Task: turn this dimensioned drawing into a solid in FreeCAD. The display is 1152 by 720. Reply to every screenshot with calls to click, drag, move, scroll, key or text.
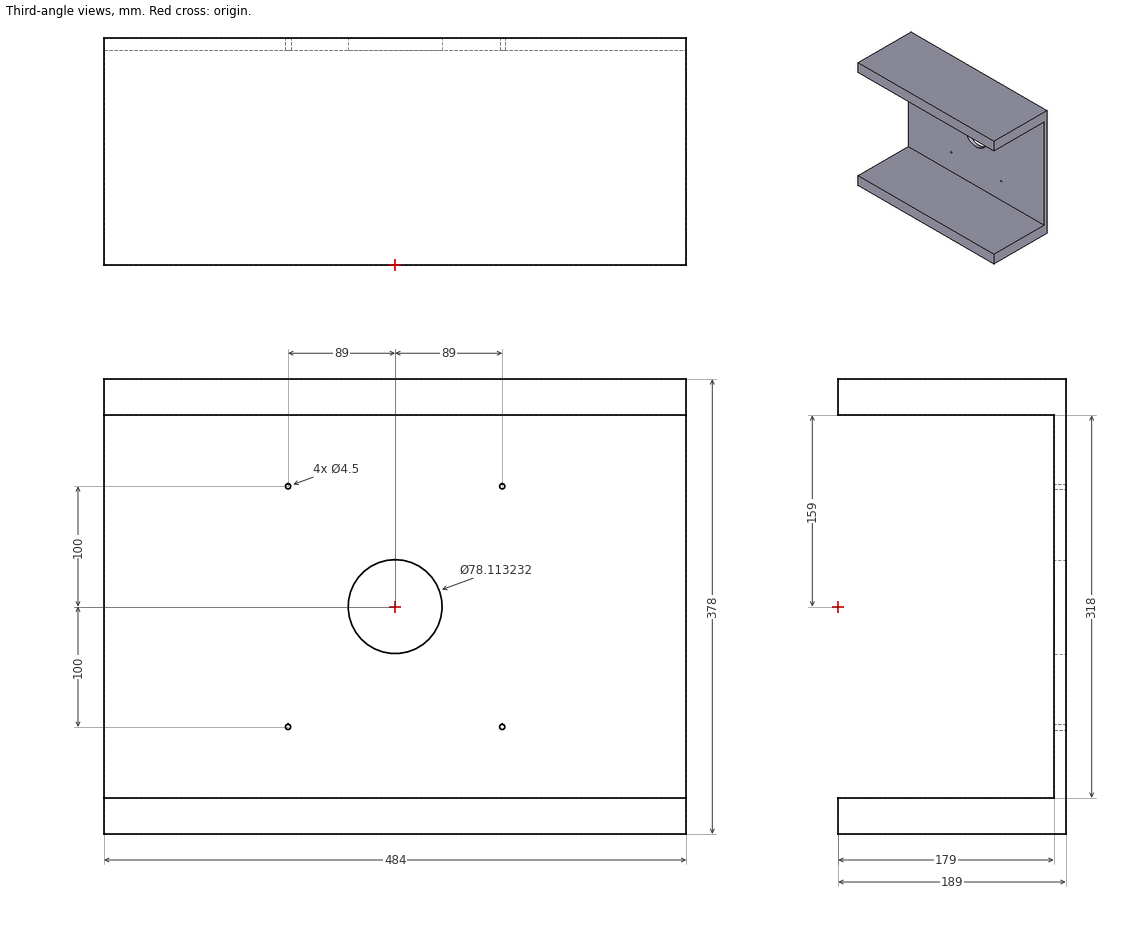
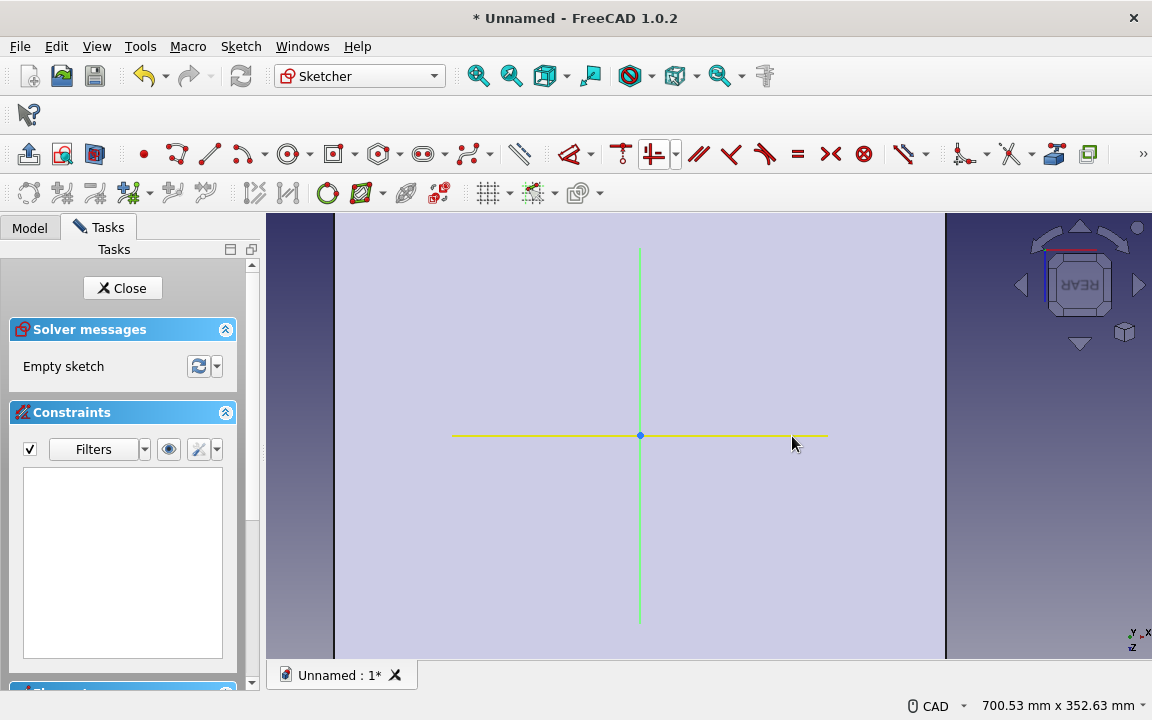
click(288, 154)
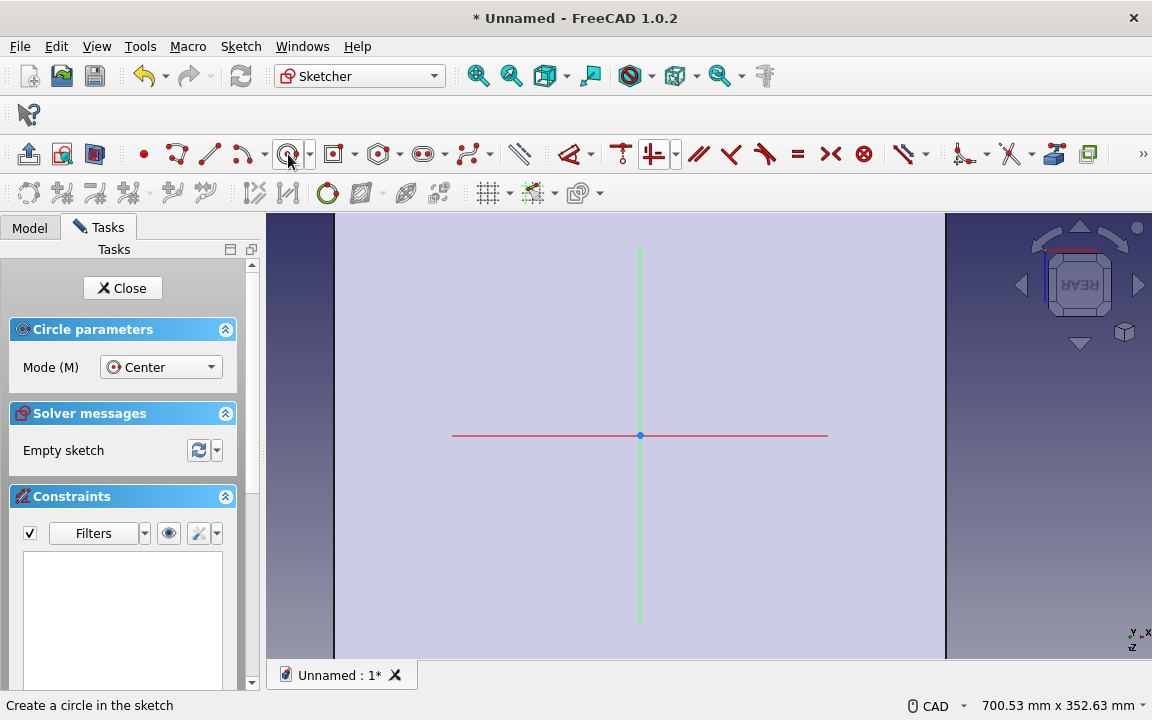
scroll(528, 562, up, 11)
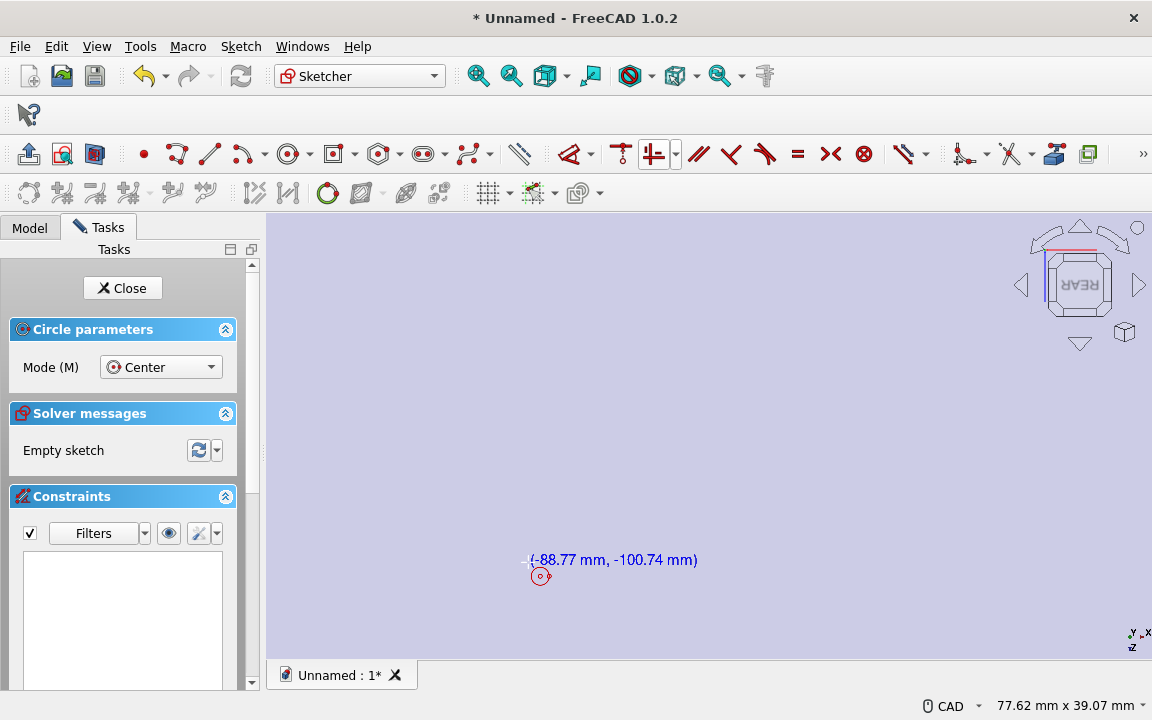
scroll(529, 563, down, 11)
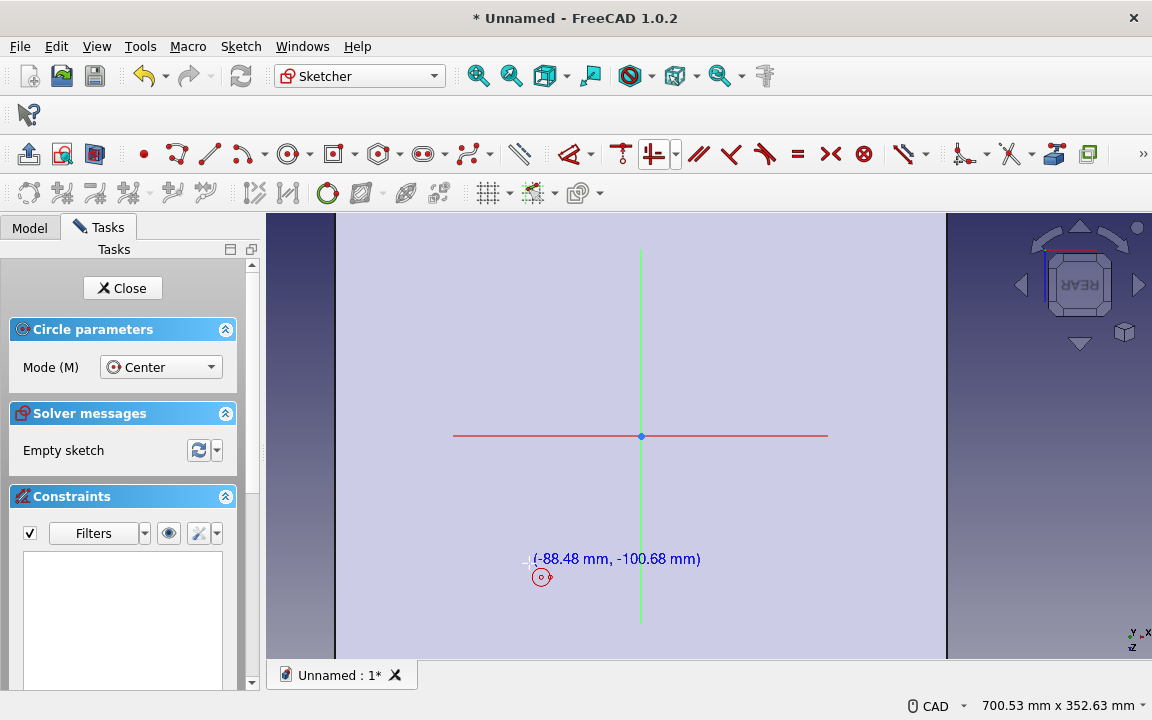
click(529, 563)
move(531, 561)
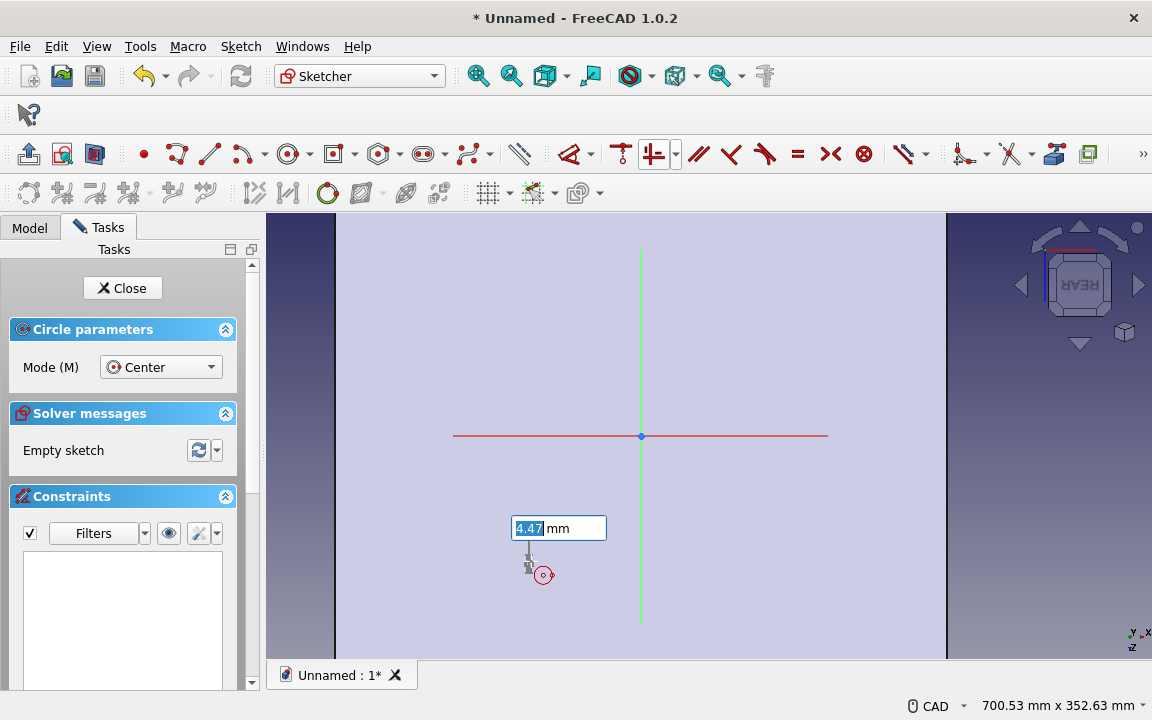
text(4.5)
key(Return)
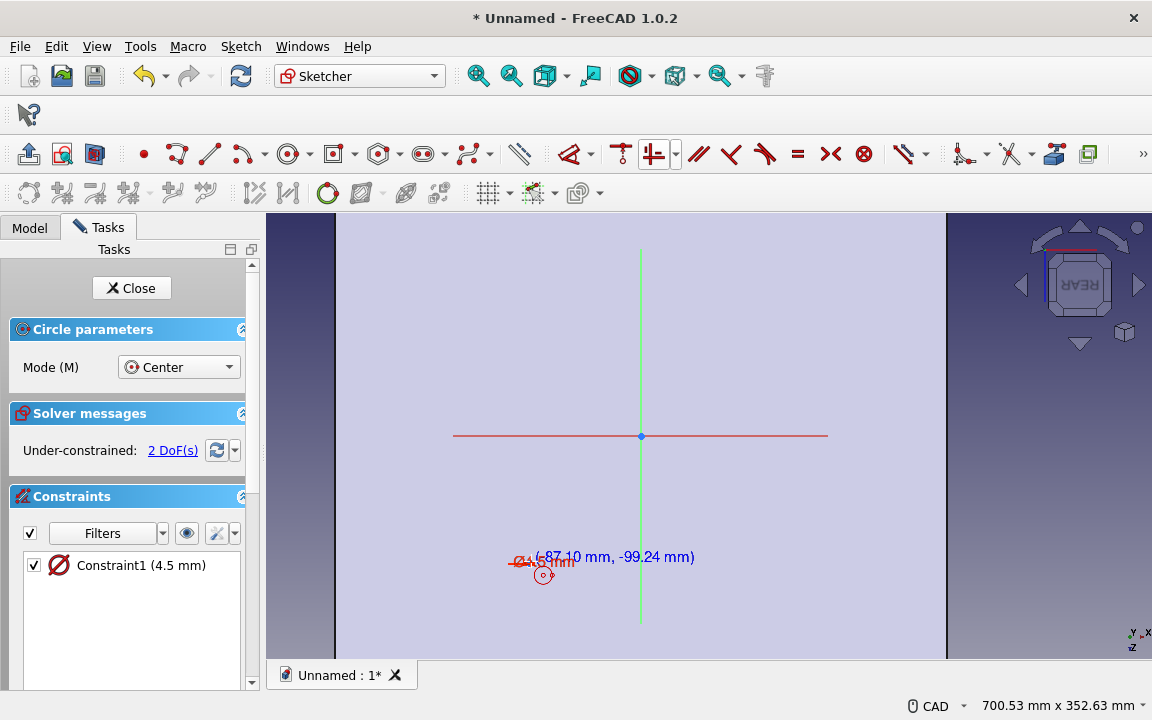
scroll(754, 563, up, 11)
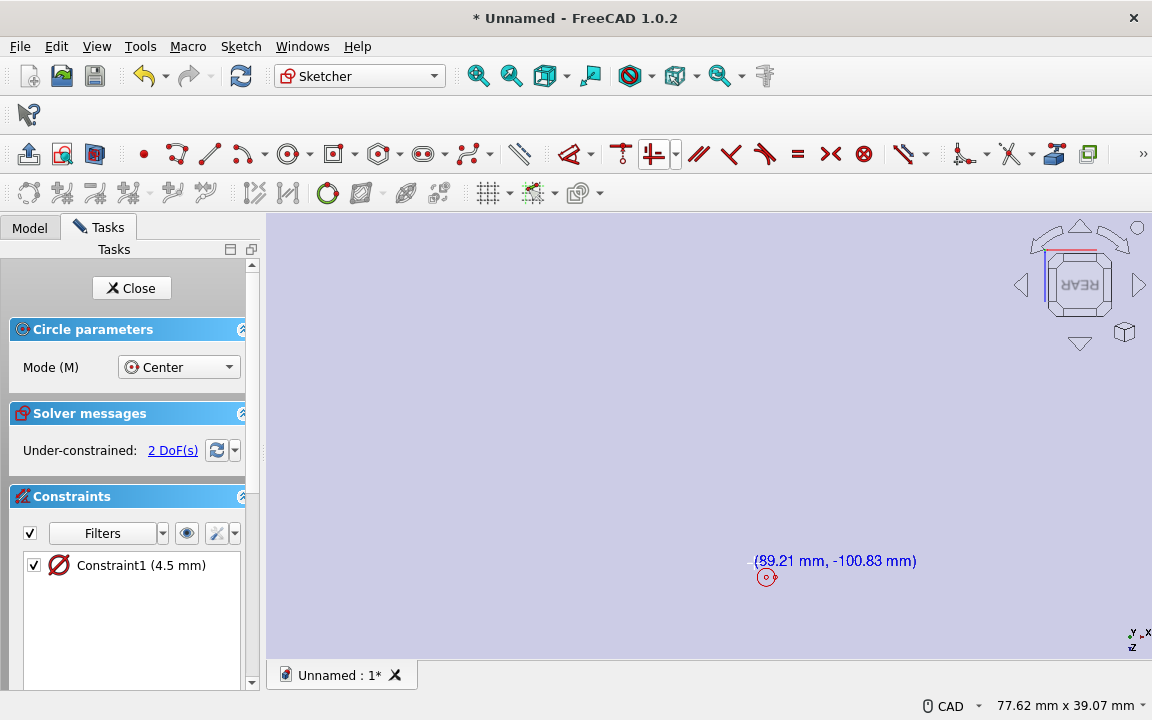
scroll(754, 563, down, 11)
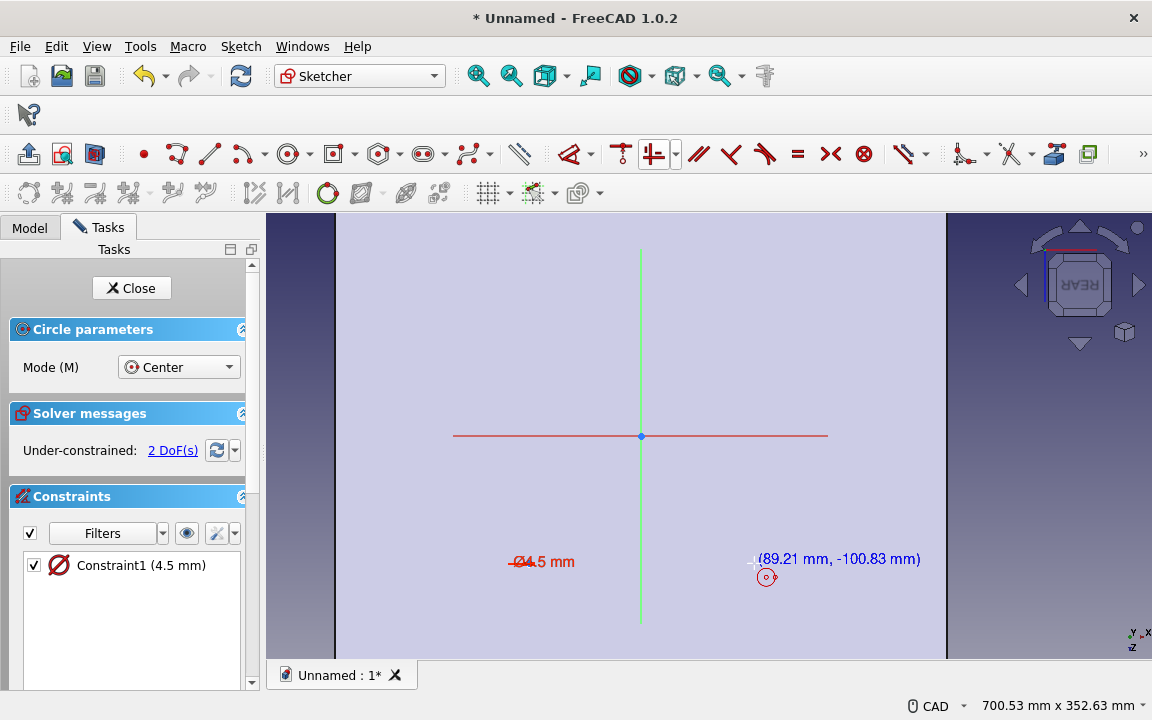
click(754, 563)
move(756, 561)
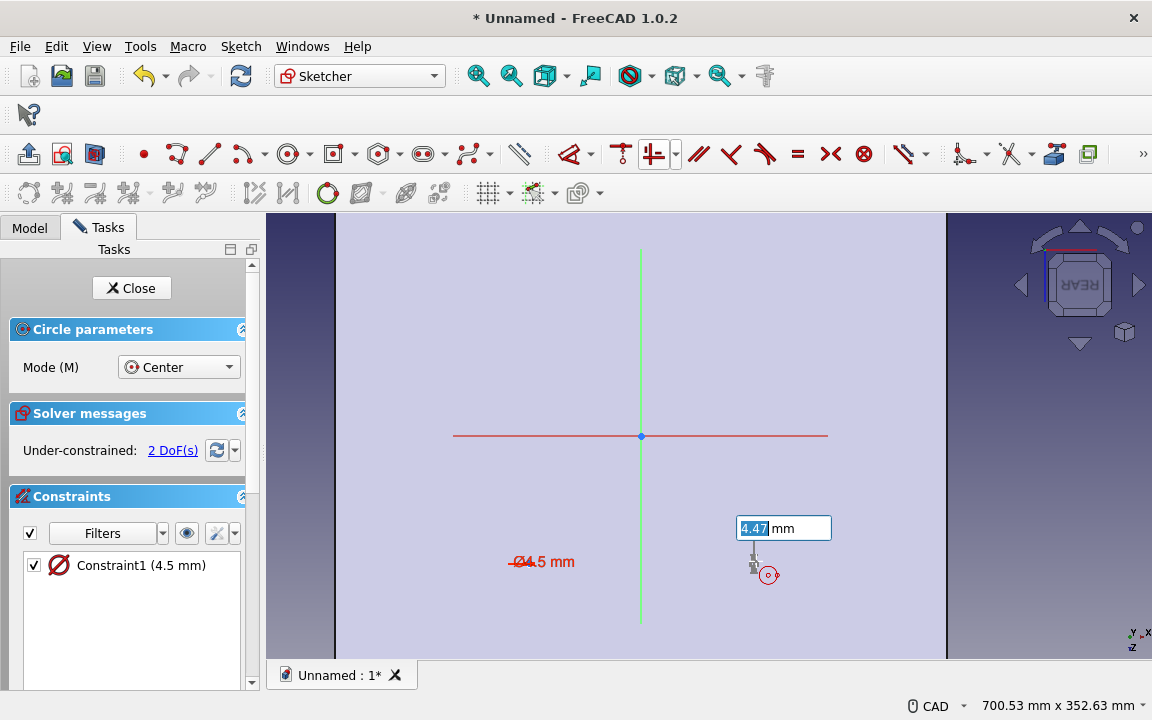
text(4.5)
key(Return)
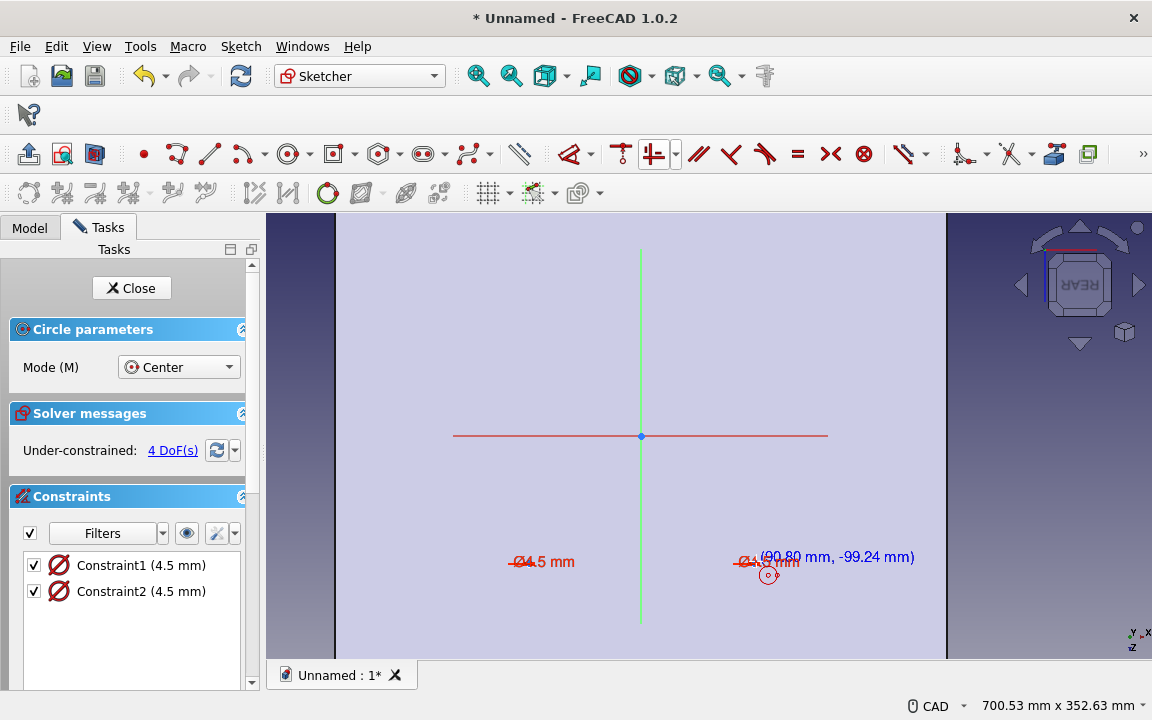
scroll(529, 310, up, 11)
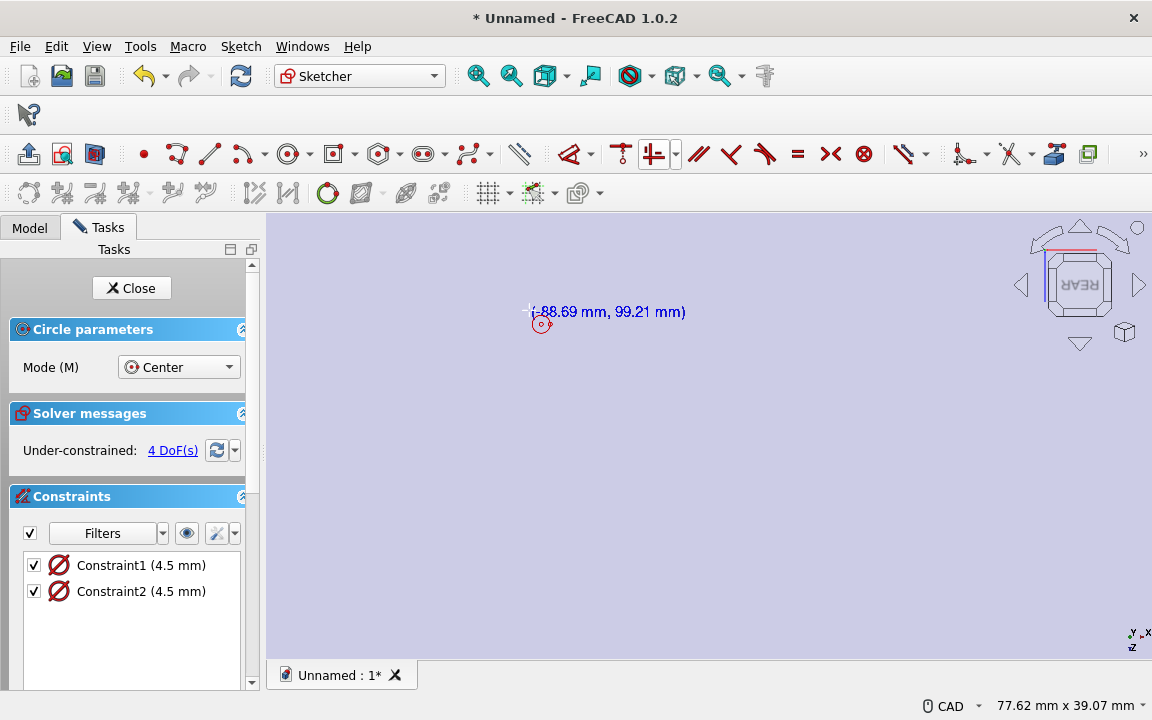
scroll(529, 310, down, 11)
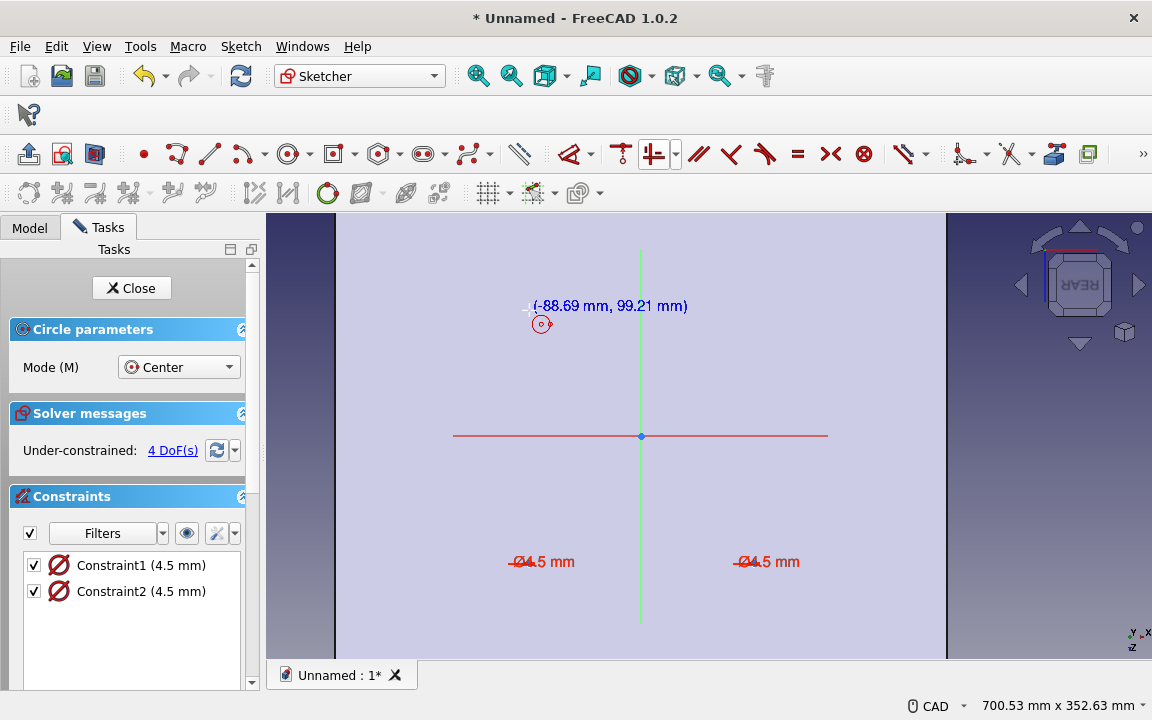
click(529, 310)
move(531, 308)